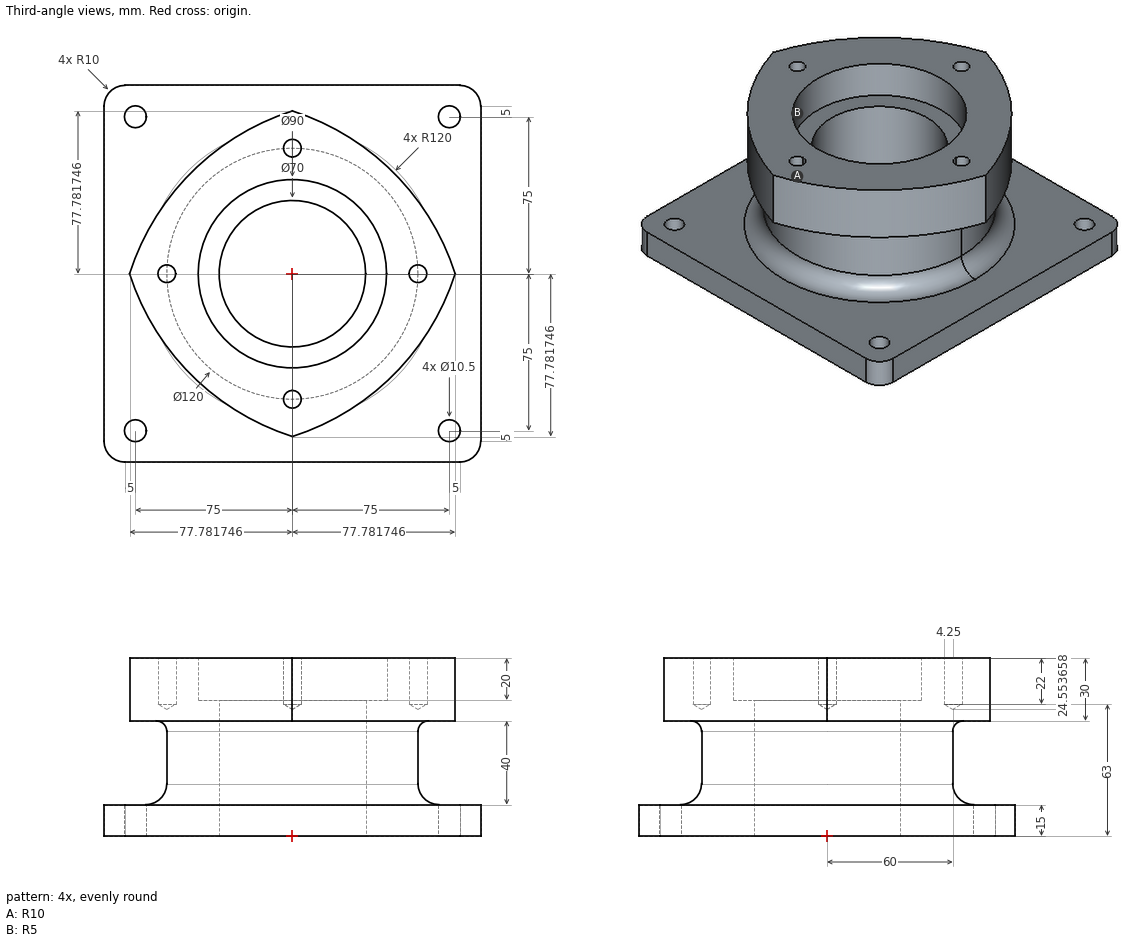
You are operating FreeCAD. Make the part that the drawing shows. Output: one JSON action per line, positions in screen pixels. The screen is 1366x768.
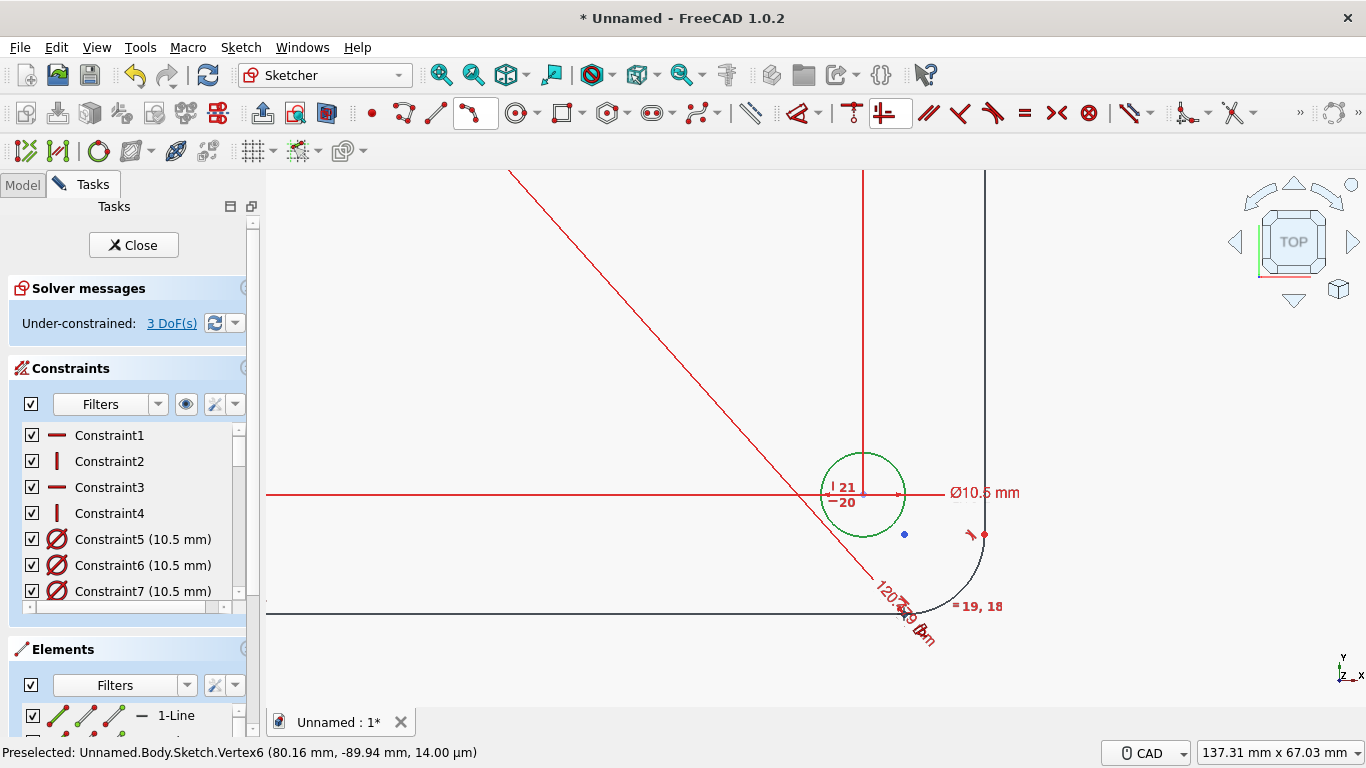
{"action": "left_click", "coordinate": [863, 495]}
{"action": "left_click", "coordinate": [884, 648]}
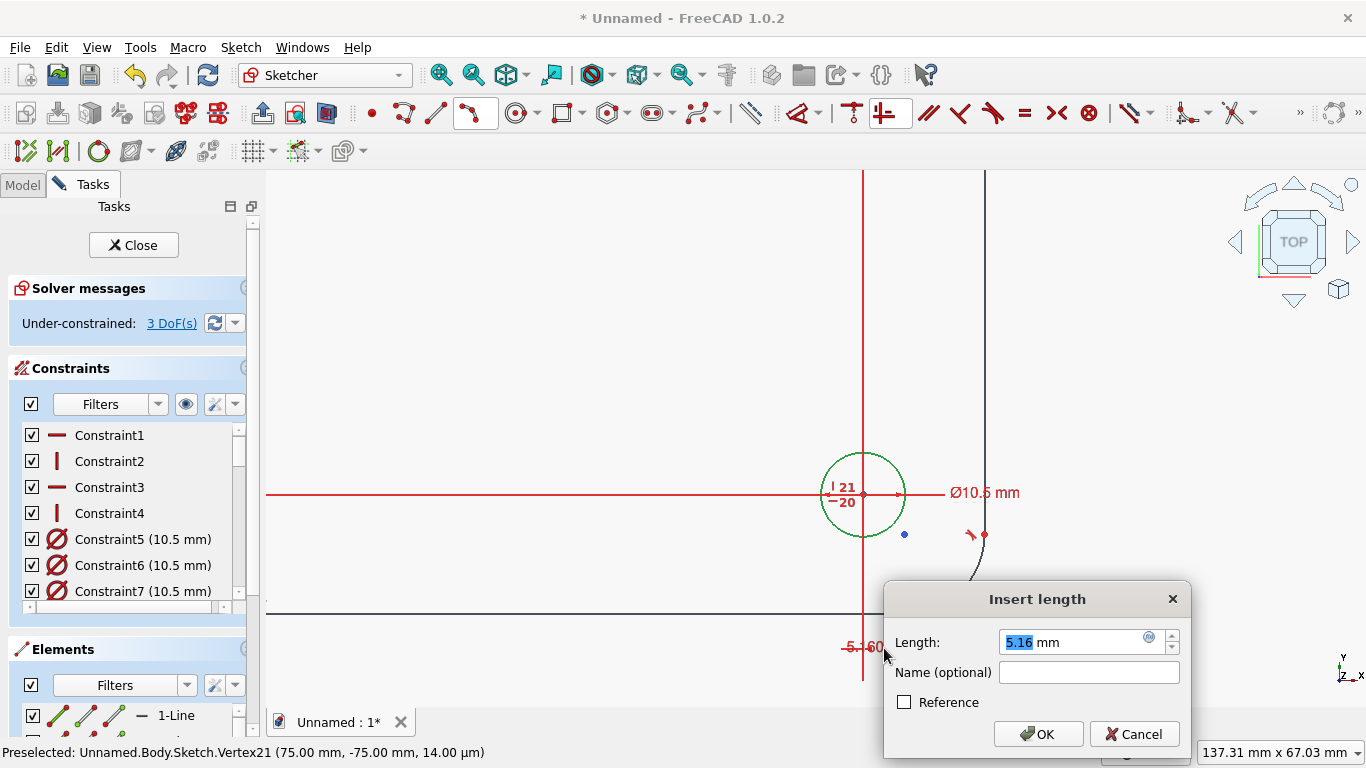
{"action": "type", "text": "5"}
{"action": "key", "text": "Return"}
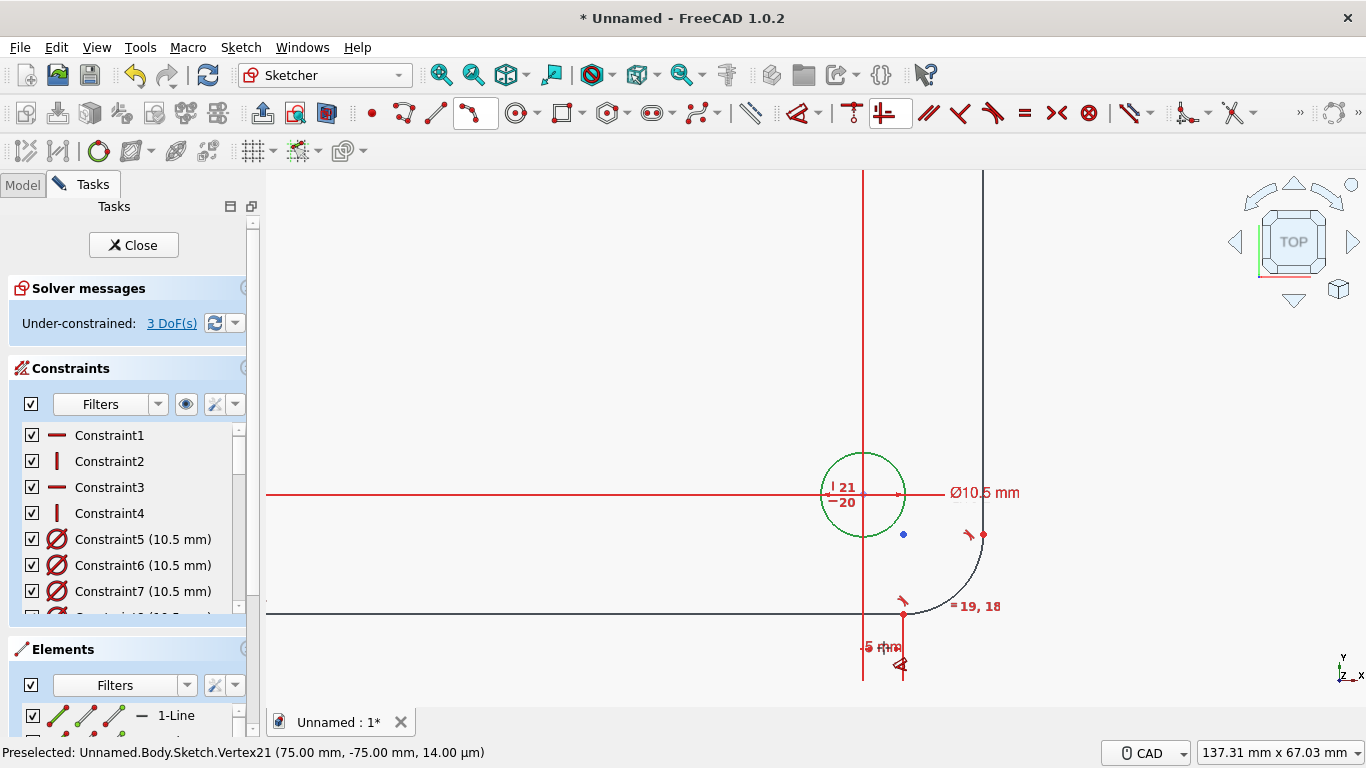
{"action": "left_click", "coordinate": [983, 534]}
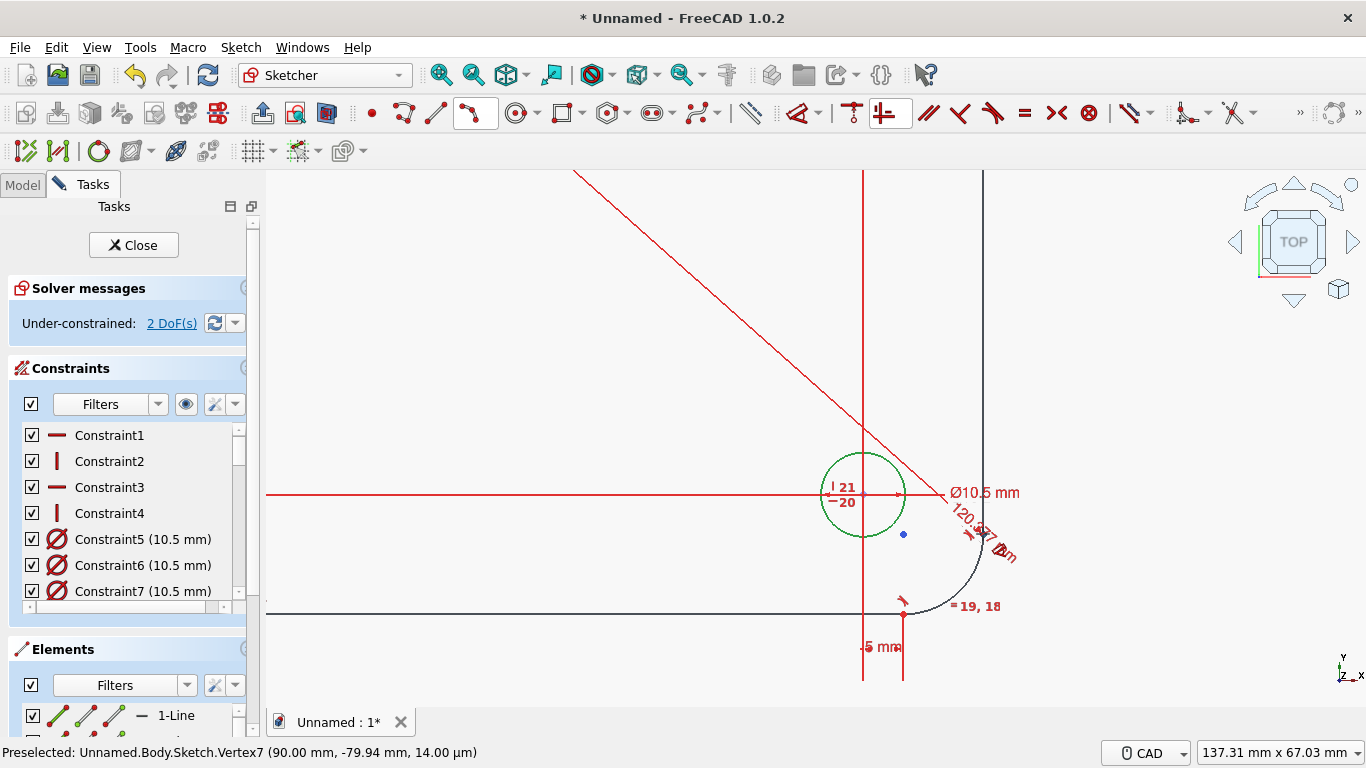
{"action": "left_click", "coordinate": [863, 495]}
{"action": "left_click", "coordinate": [1017, 514]}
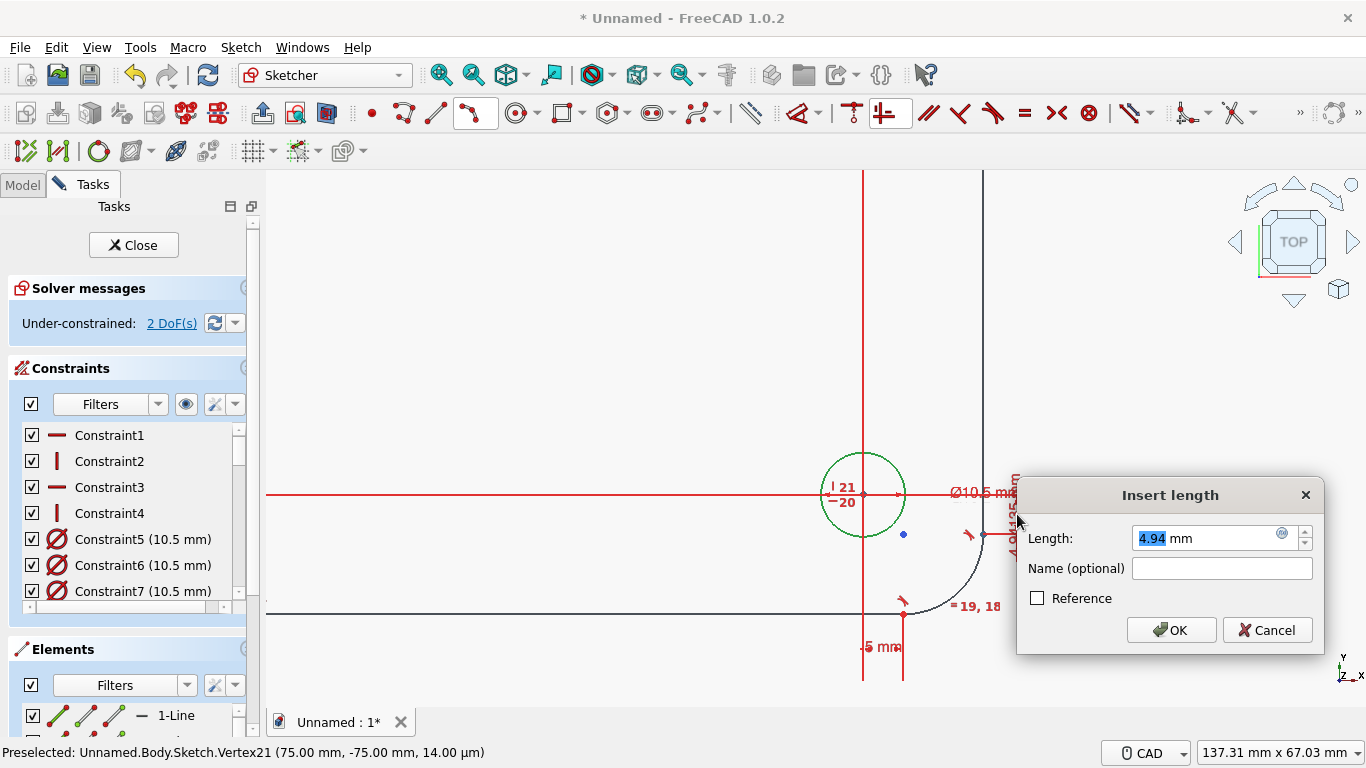
{"action": "type", "text": "5"}
{"action": "key", "text": "Return"}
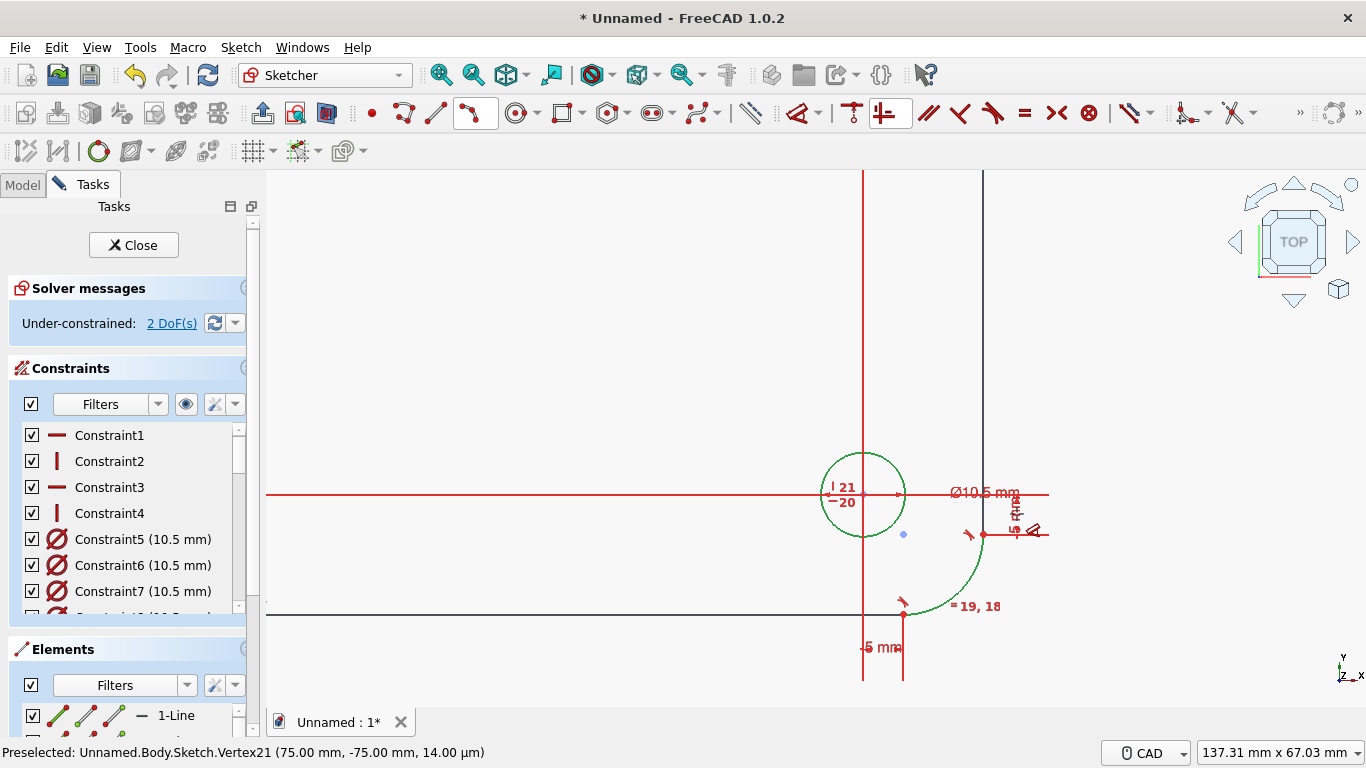
{"action": "scroll", "coordinate": [906, 617], "scroll_direction": "down", "scroll_amount": 7}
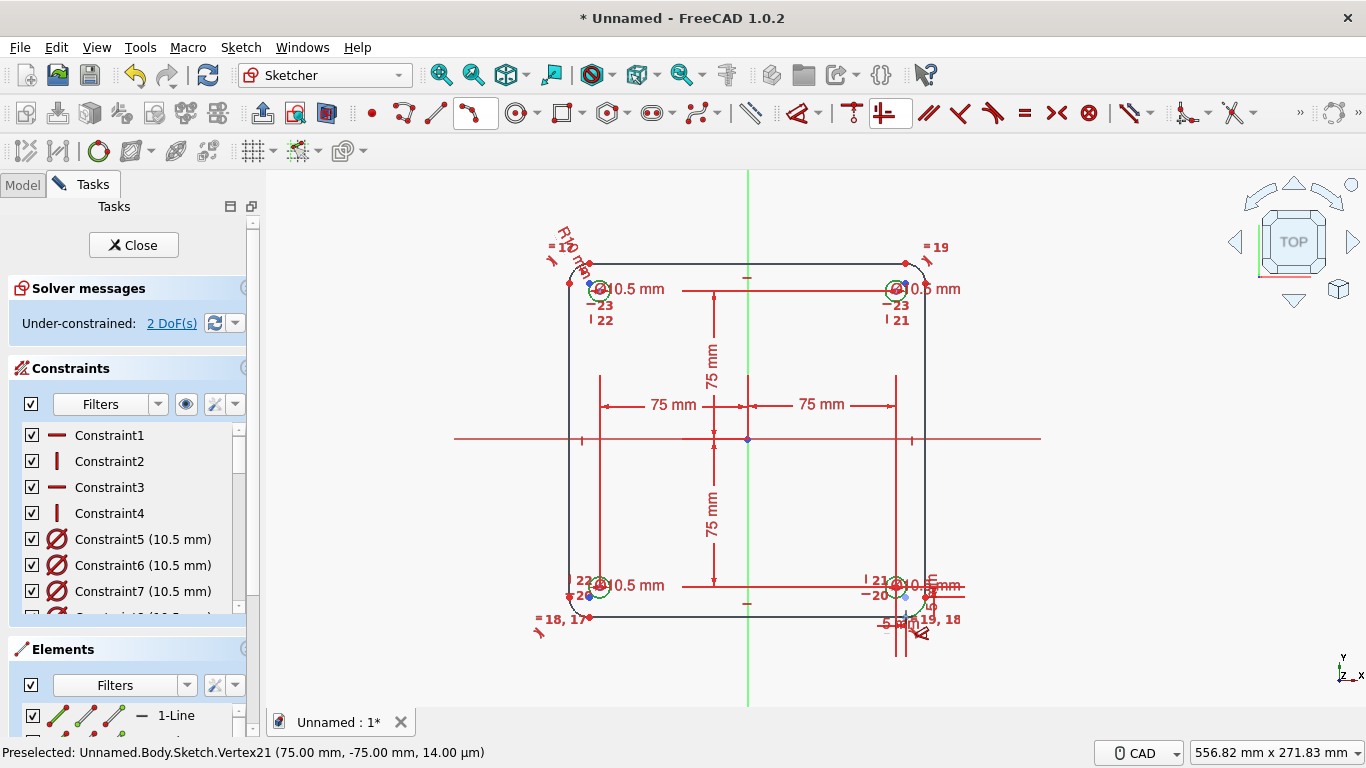
{"action": "scroll", "coordinate": [589, 617], "scroll_direction": "up", "scroll_amount": 7}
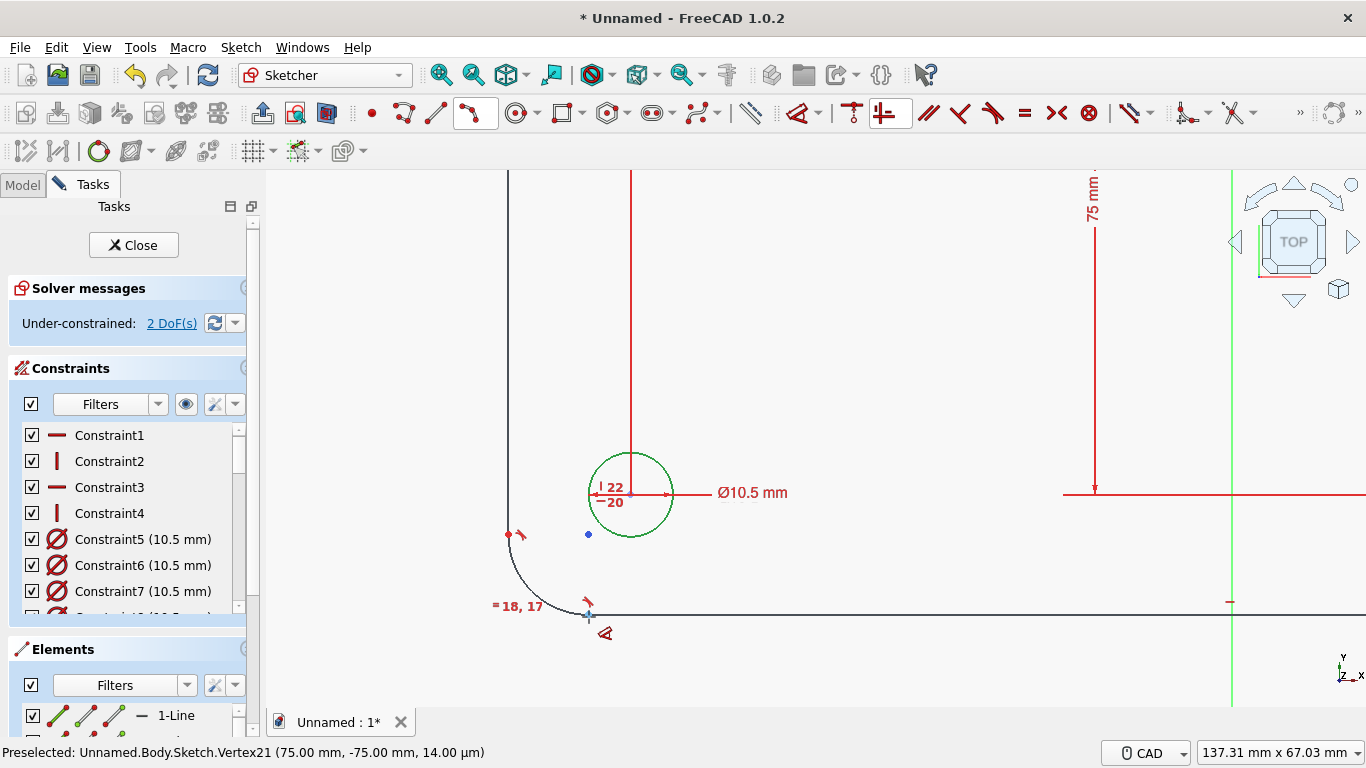
{"action": "left_click", "coordinate": [589, 615]}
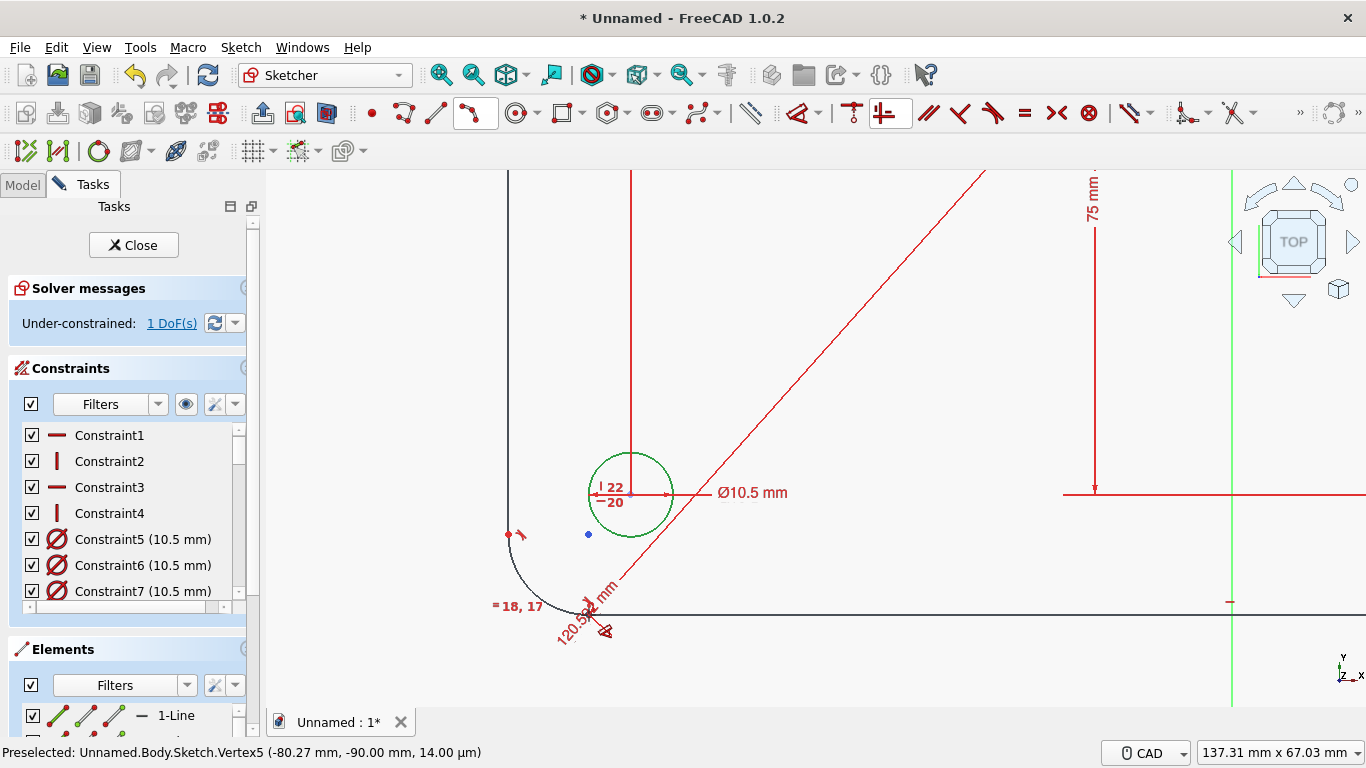
{"action": "left_click", "coordinate": [631, 495]}
{"action": "left_click", "coordinate": [610, 649]}